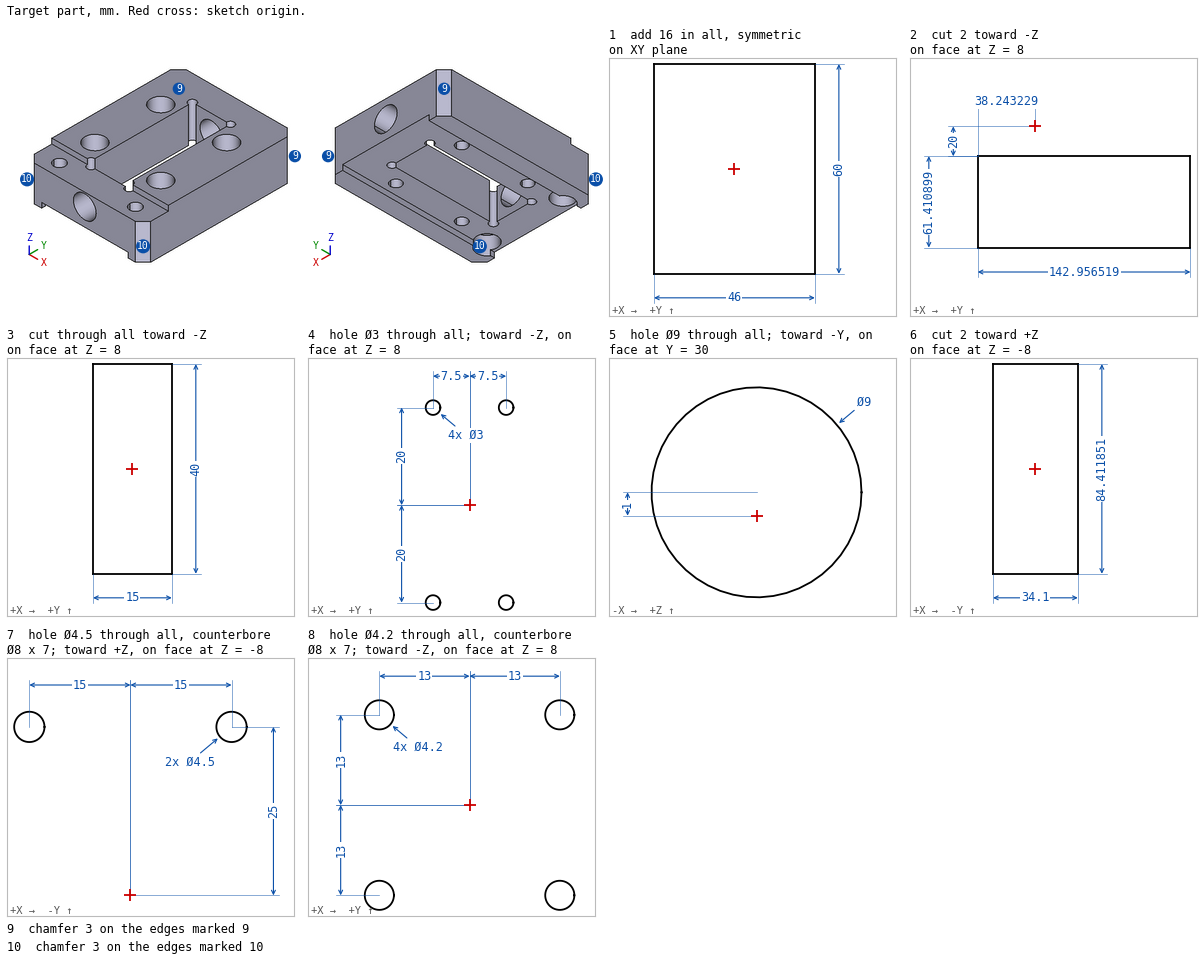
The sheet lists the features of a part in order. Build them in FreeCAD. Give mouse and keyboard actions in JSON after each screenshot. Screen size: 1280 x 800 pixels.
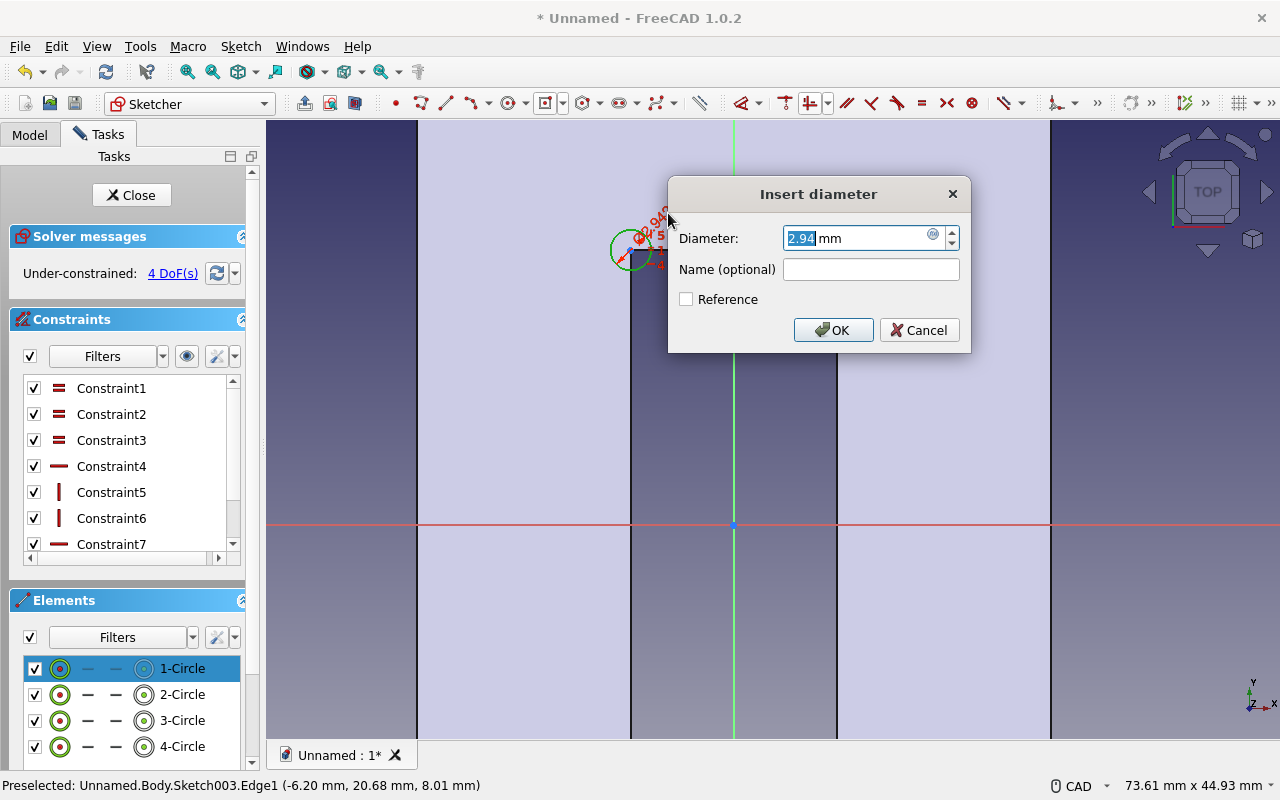
{"action": "type", "text": "3"}
{"action": "key", "text": "Return"}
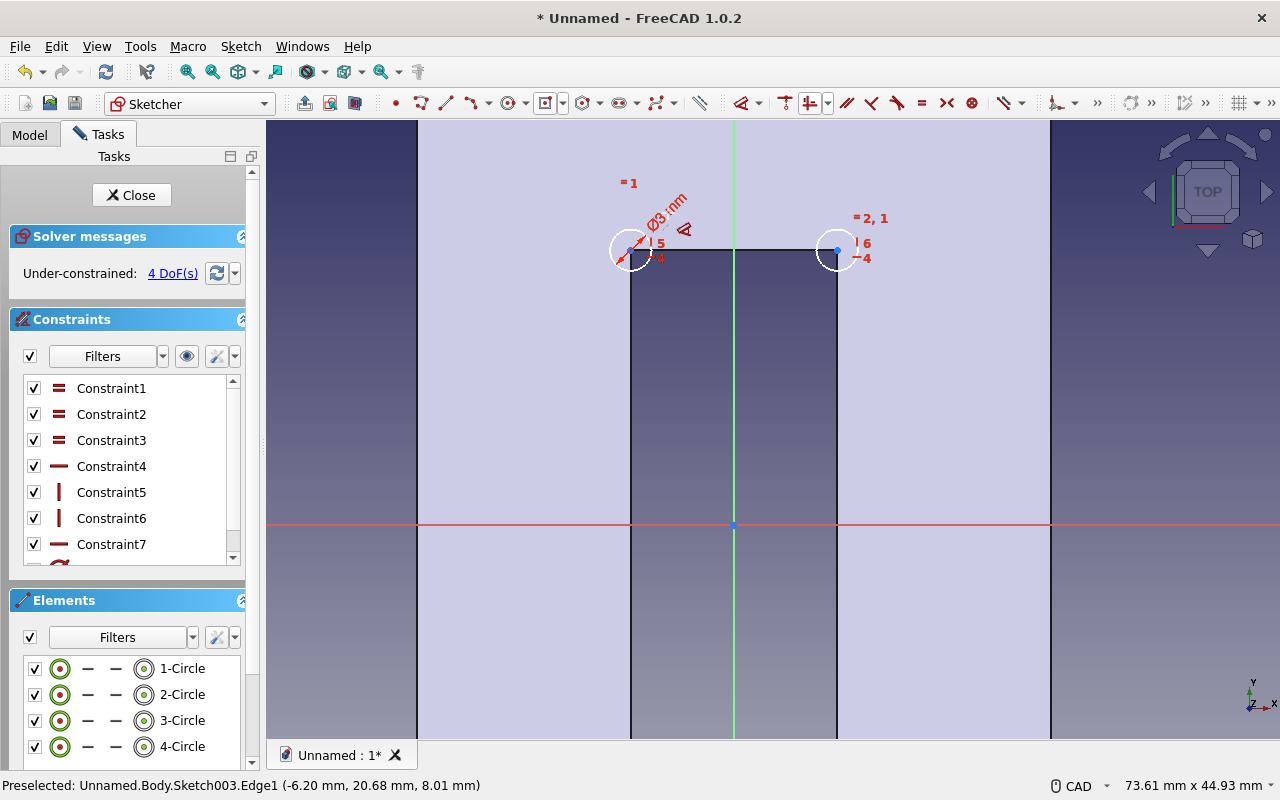
{"action": "left_click", "coordinate": [631, 250]}
{"action": "left_click", "coordinate": [597, 388]}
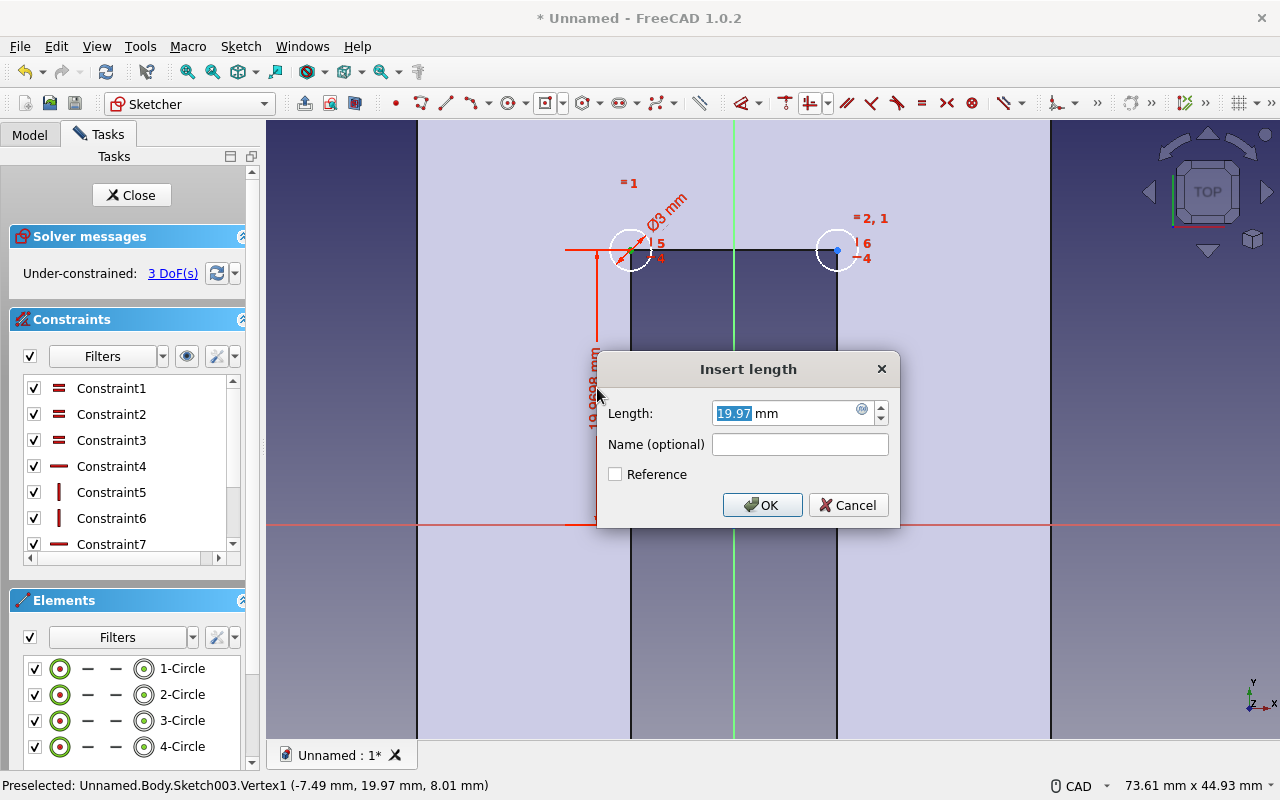
{"action": "type", "text": "20"}
{"action": "key", "text": "Return"}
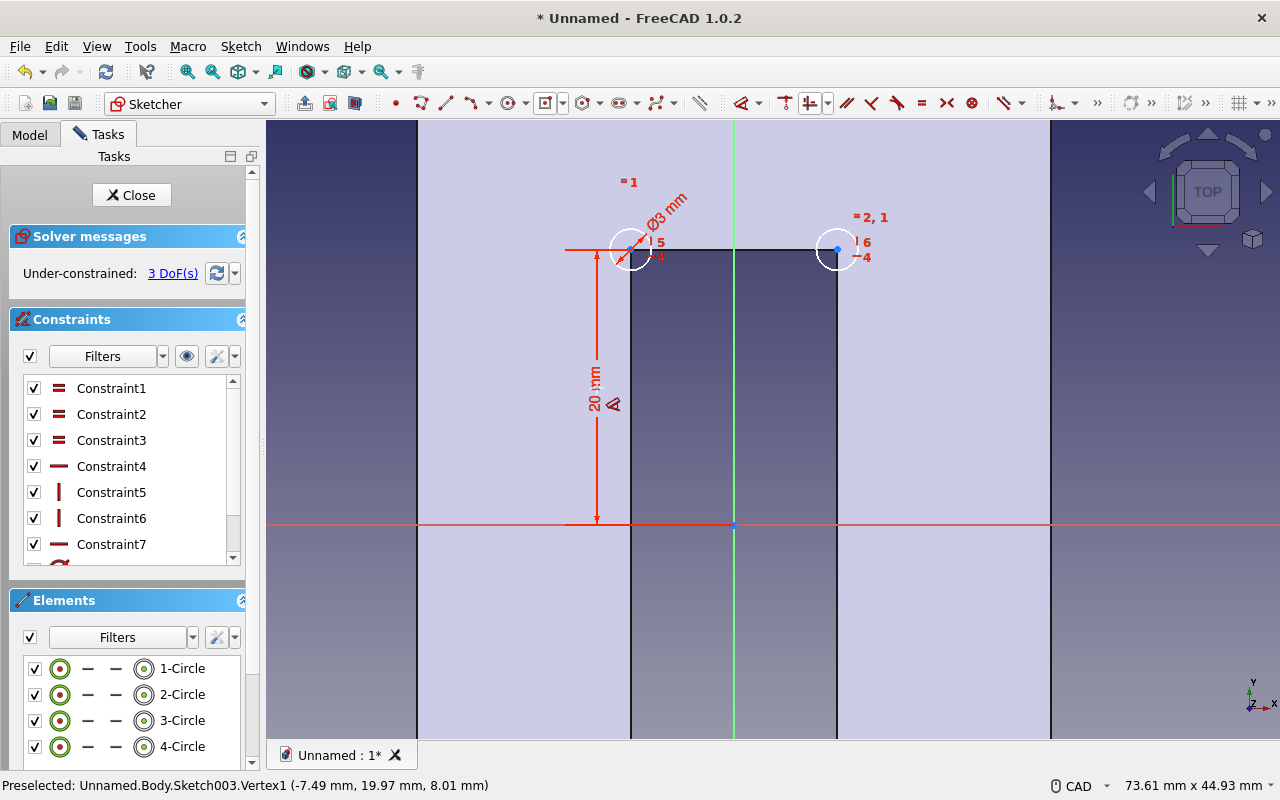
{"action": "scroll", "coordinate": [645, 235], "scroll_direction": "down", "scroll_amount": 2}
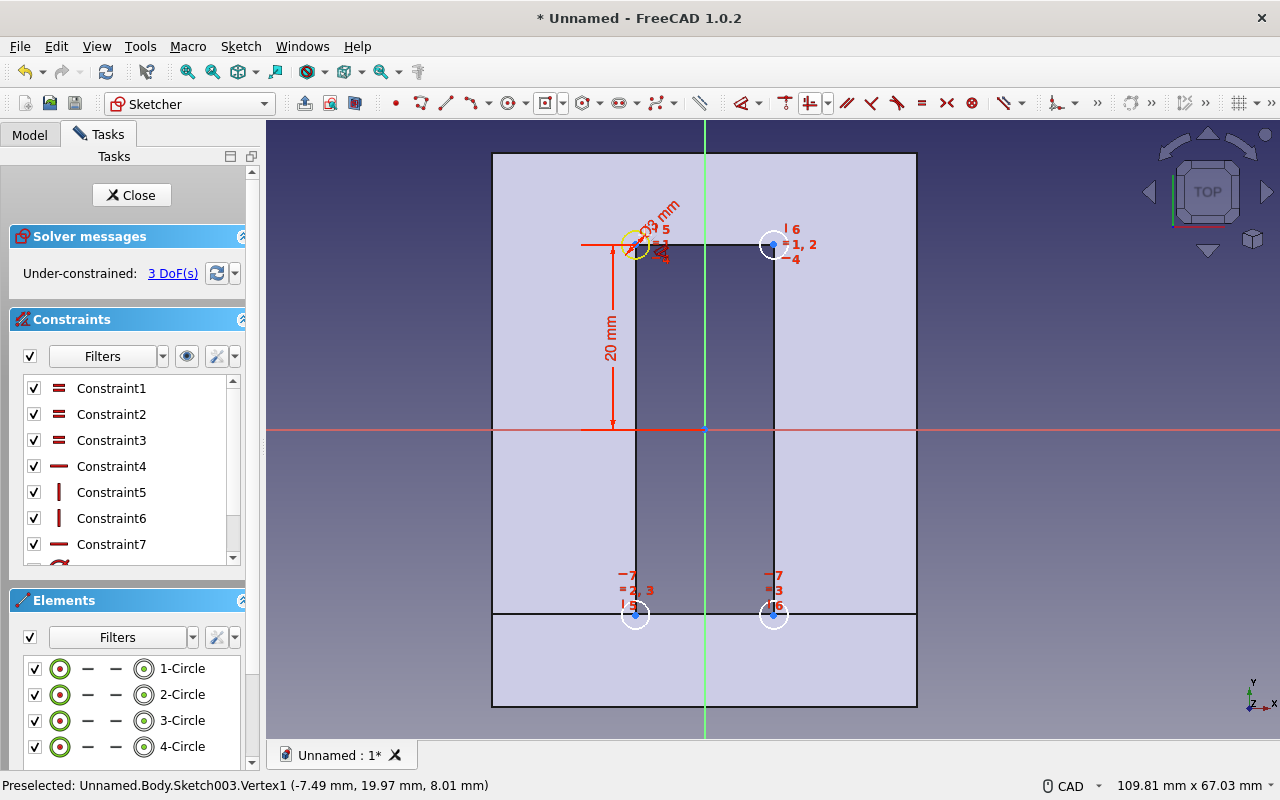
{"action": "left_click", "coordinate": [636, 615]}
{"action": "left_click", "coordinate": [602, 522]}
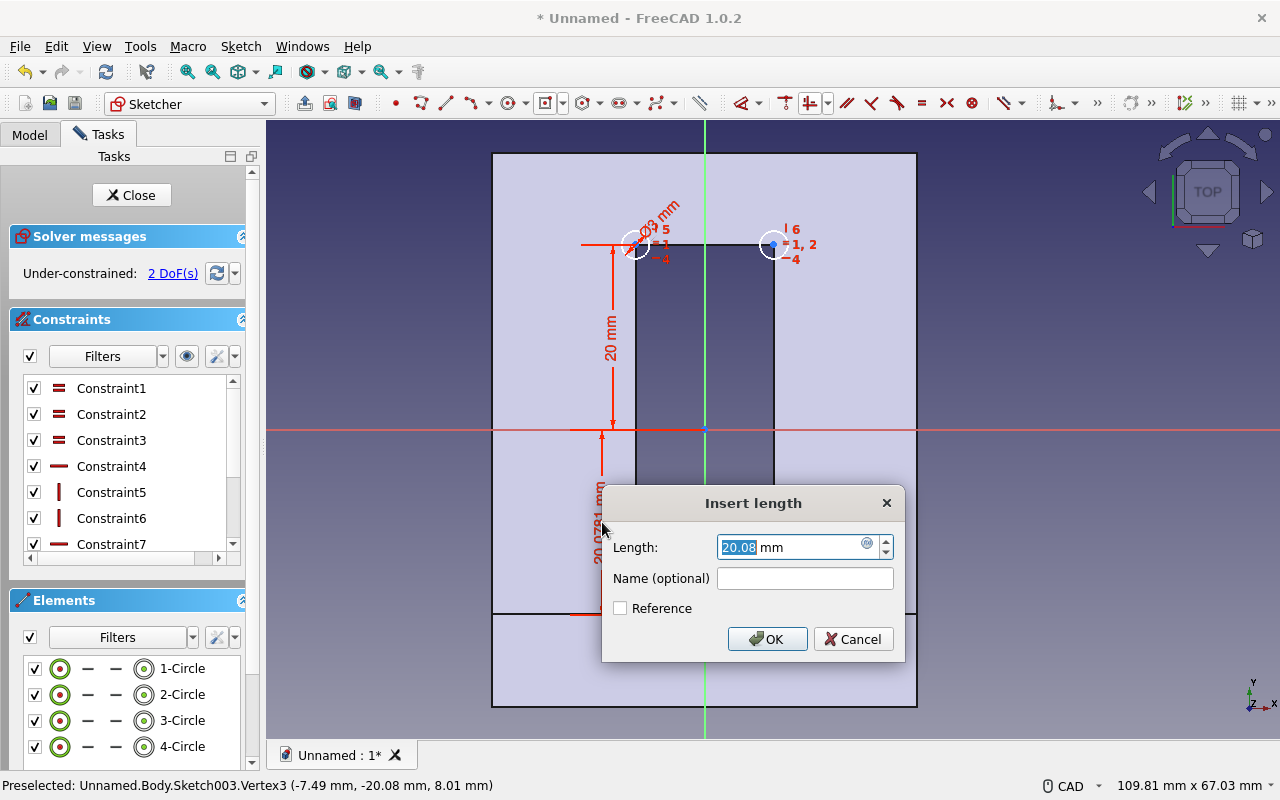
{"action": "type", "text": "20"}
{"action": "key", "text": "Return"}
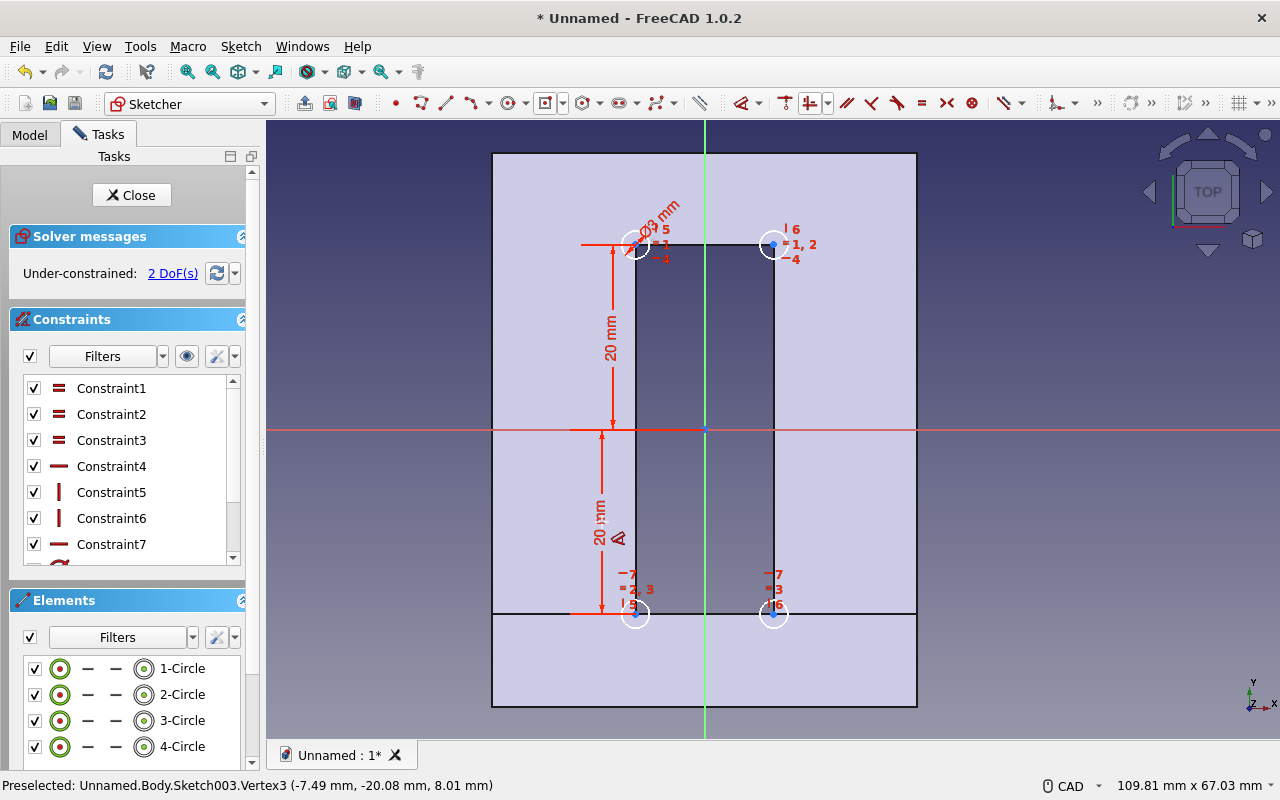
{"action": "left_click", "coordinate": [636, 245]}
{"action": "left_click", "coordinate": [670, 464]}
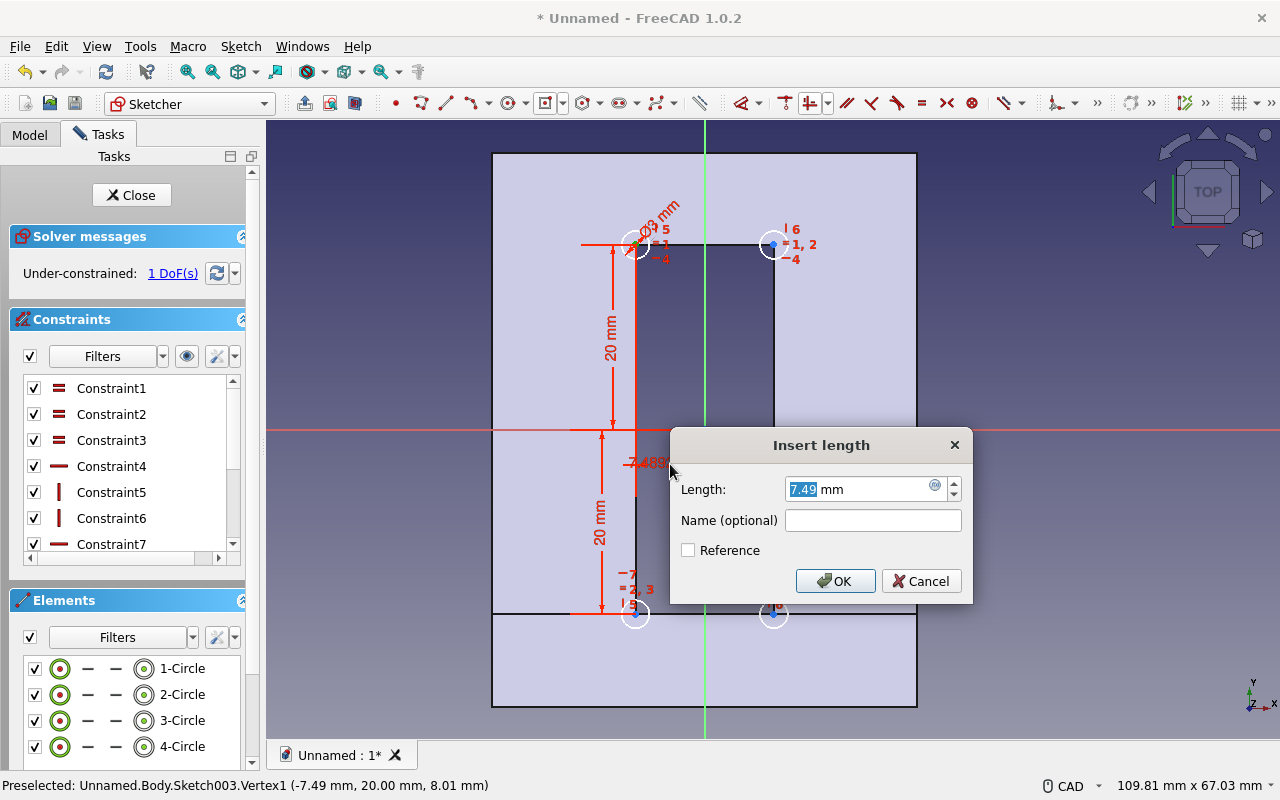
{"action": "type", "text": "7.5"}
{"action": "key", "text": "Return"}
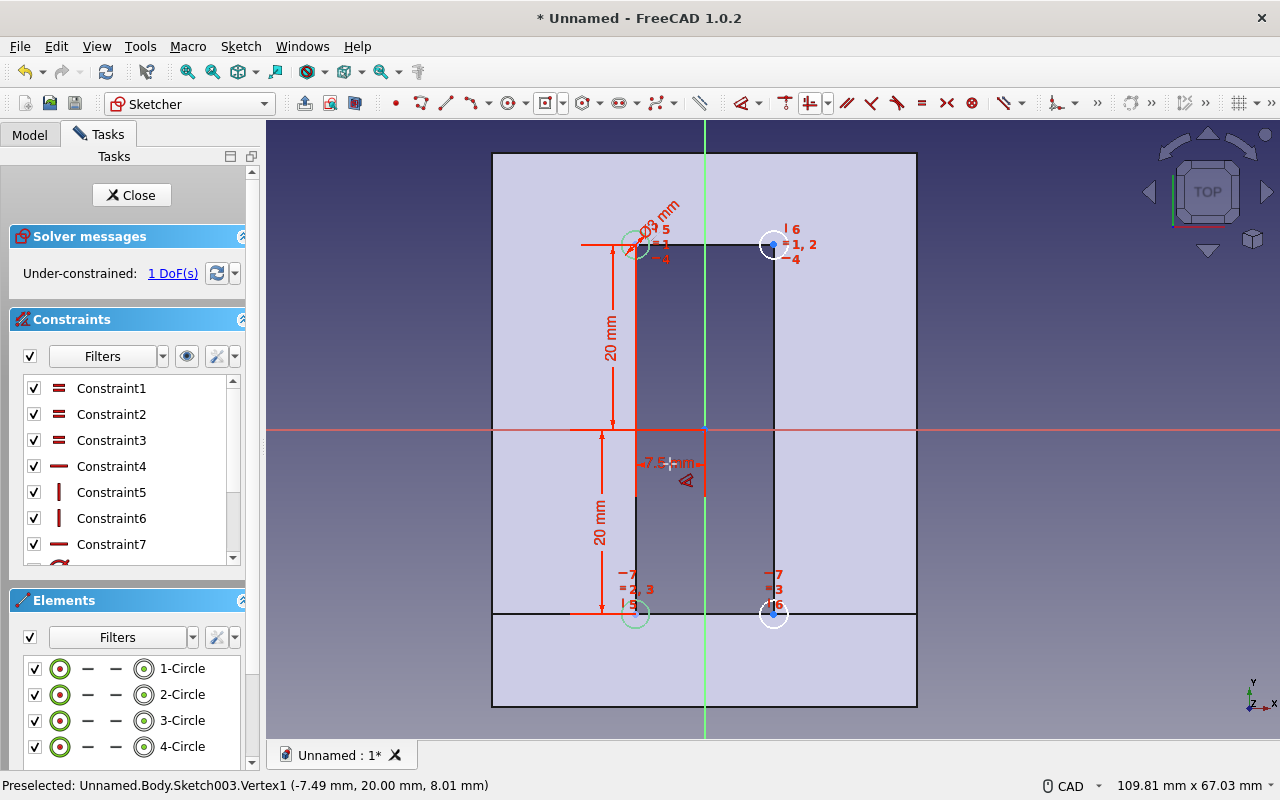
{"action": "left_click", "coordinate": [774, 245]}
{"action": "left_click", "coordinate": [739, 211]}